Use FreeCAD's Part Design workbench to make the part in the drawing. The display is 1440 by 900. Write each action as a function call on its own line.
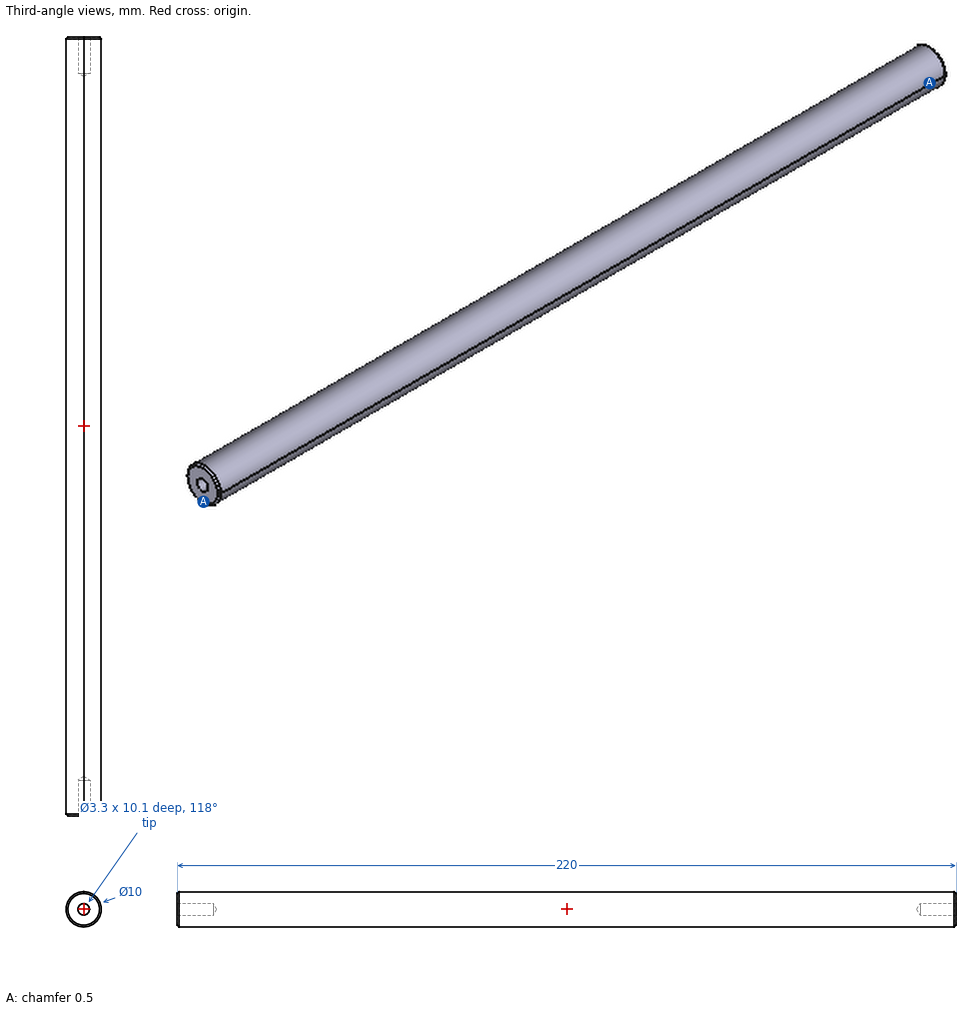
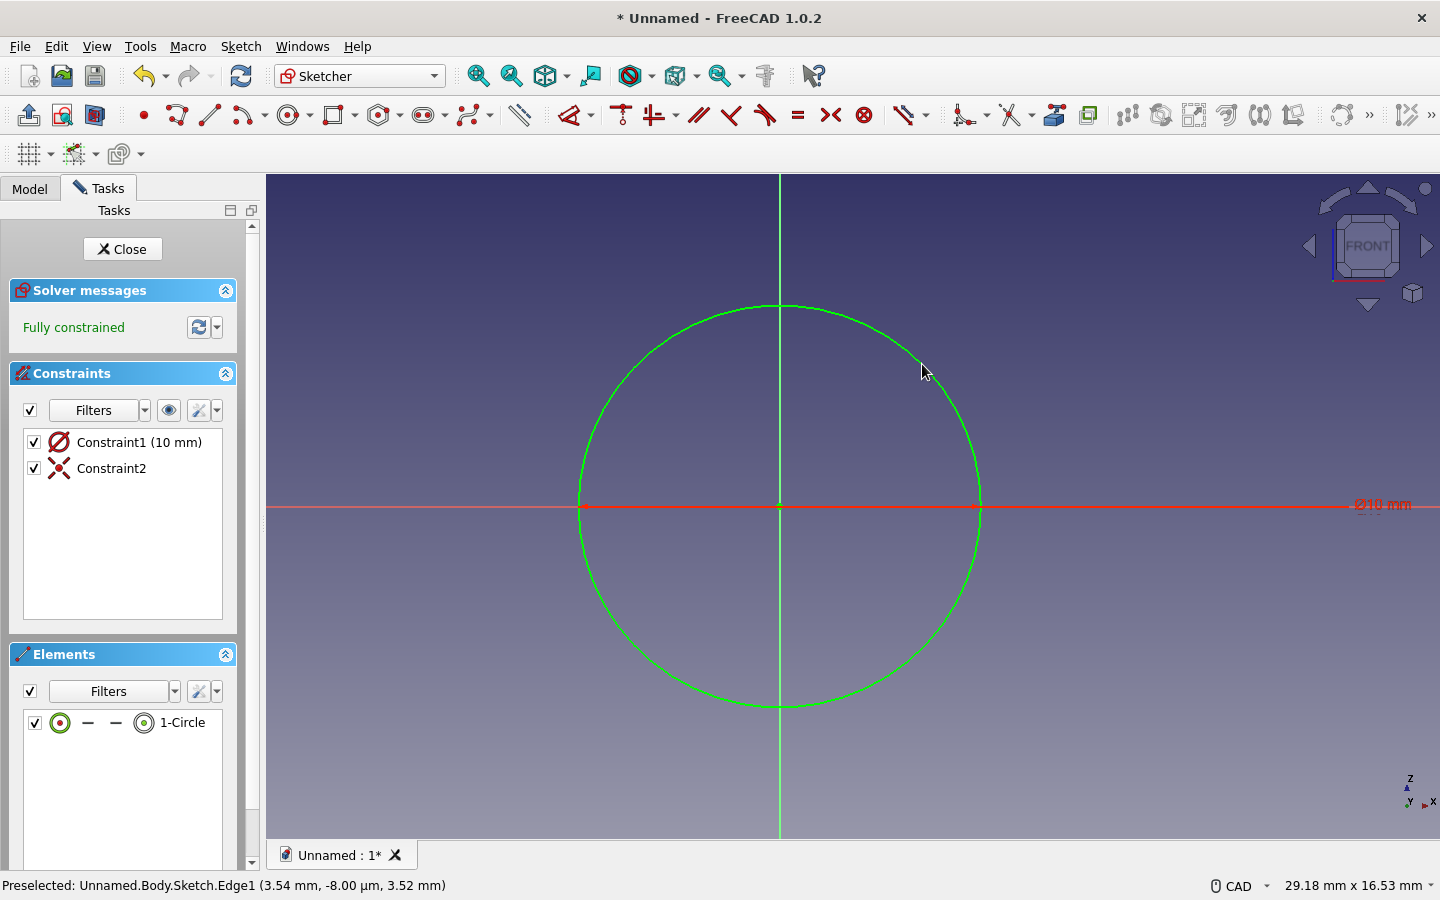
click(123, 249)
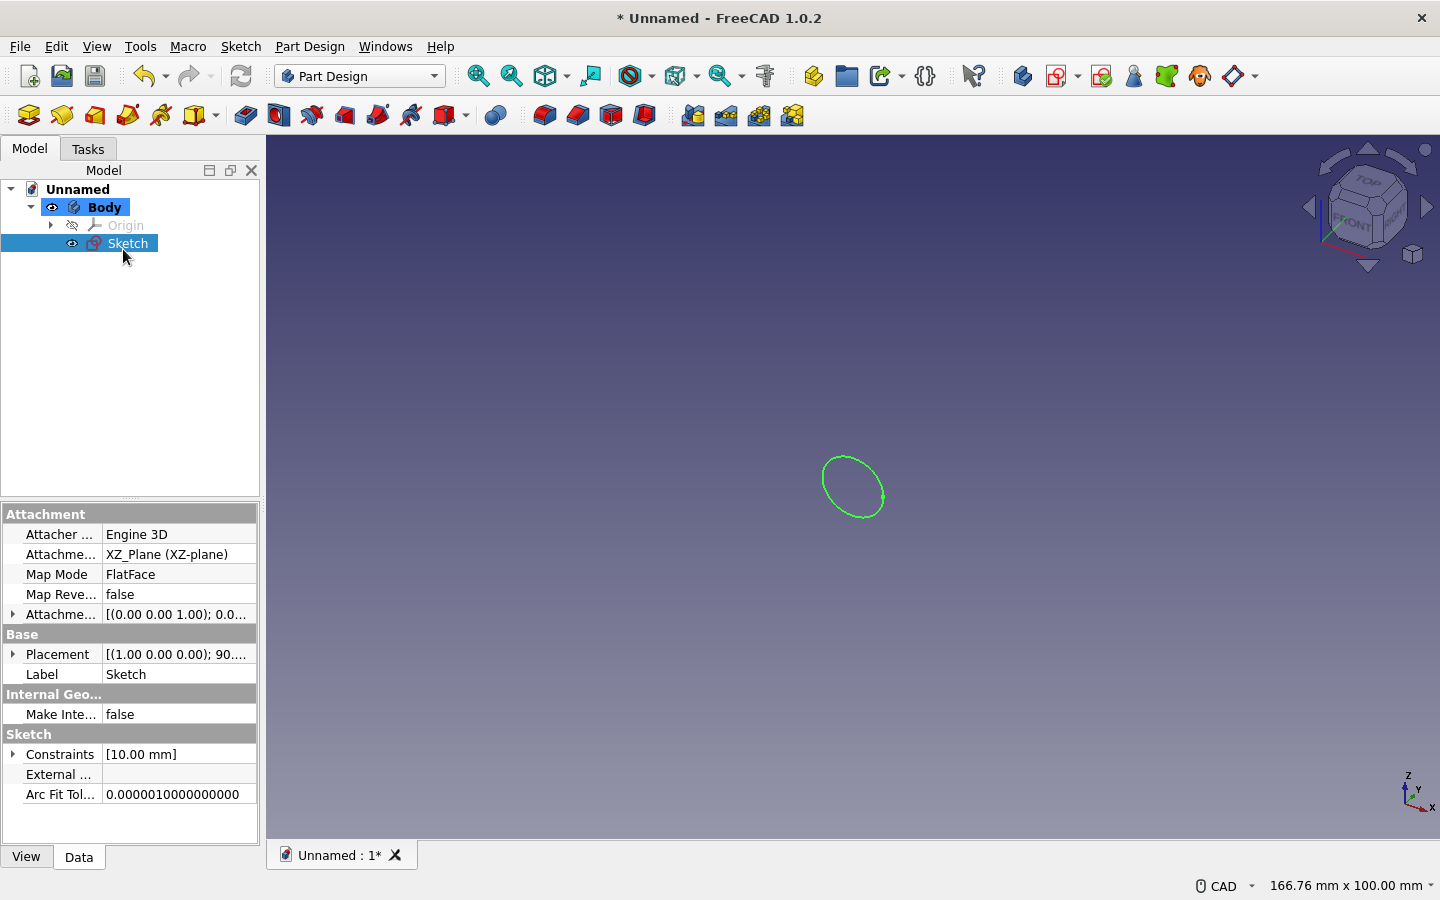
click(29, 116)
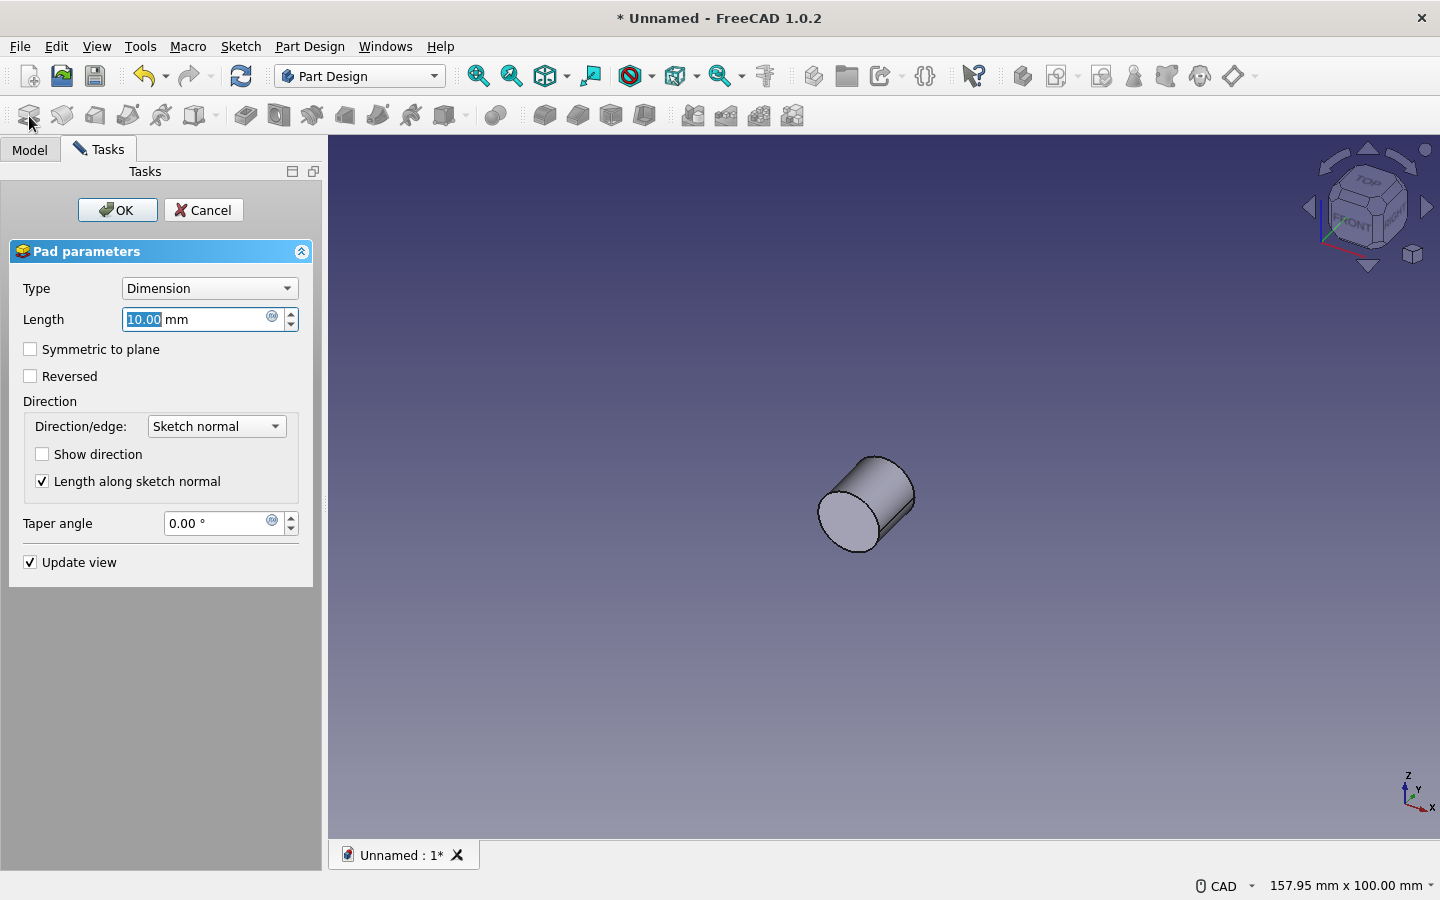
text(220)
key(Tab)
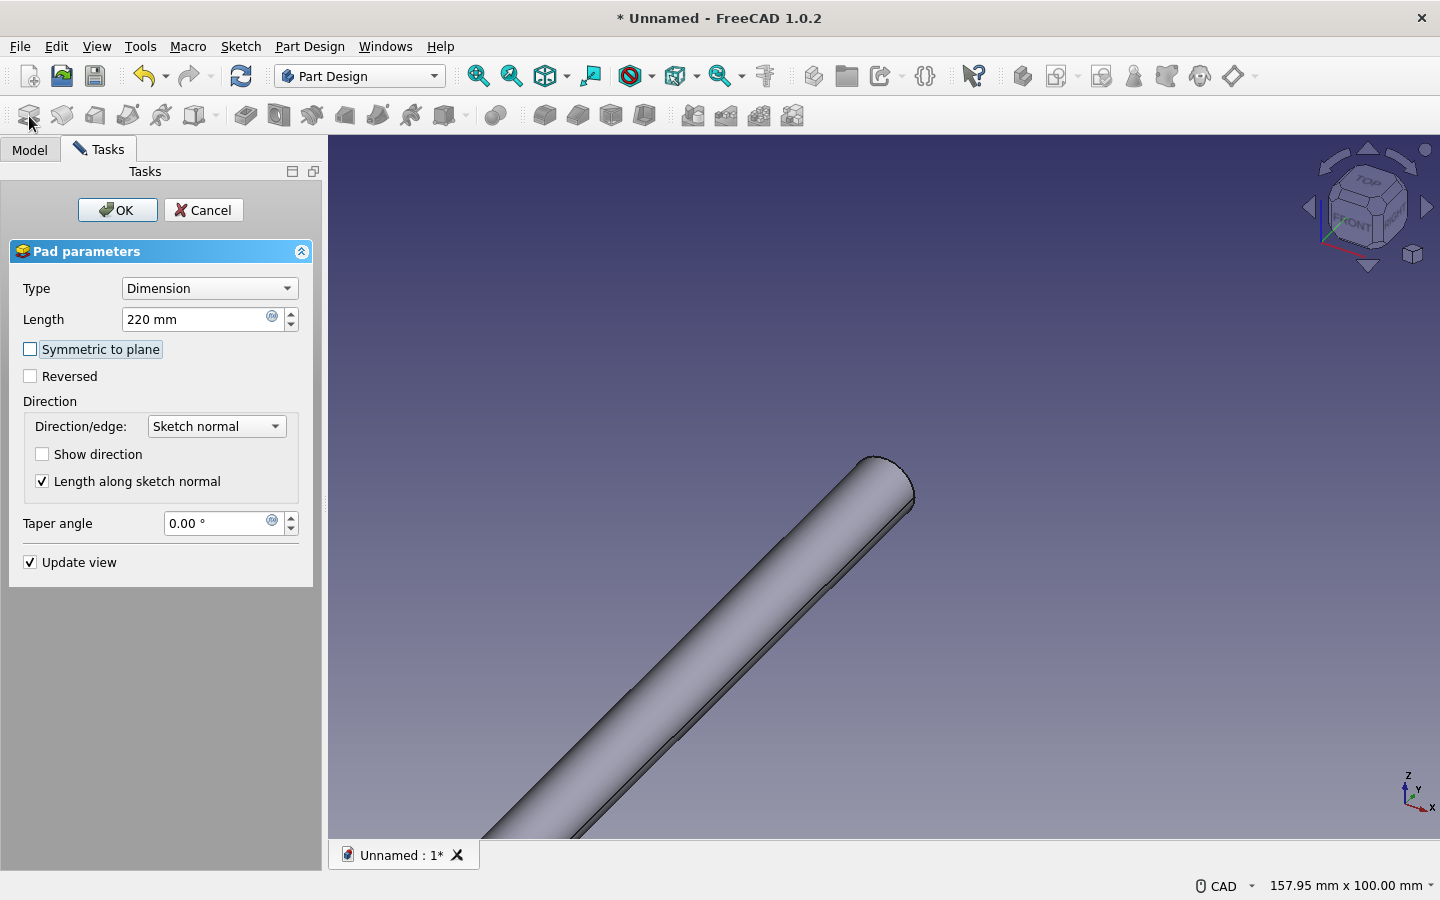
click(31, 349)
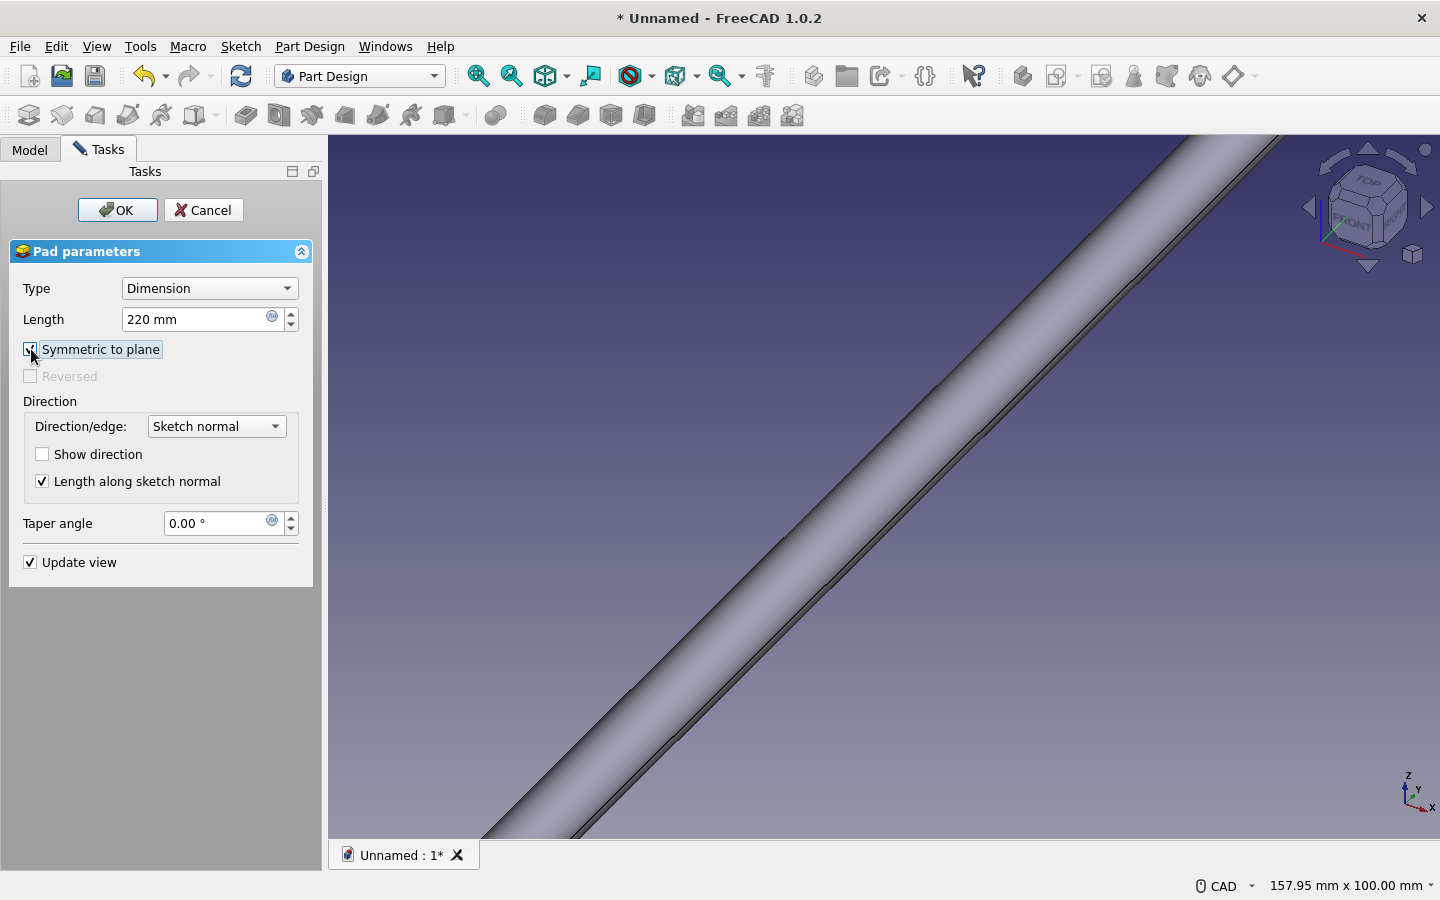
click(118, 210)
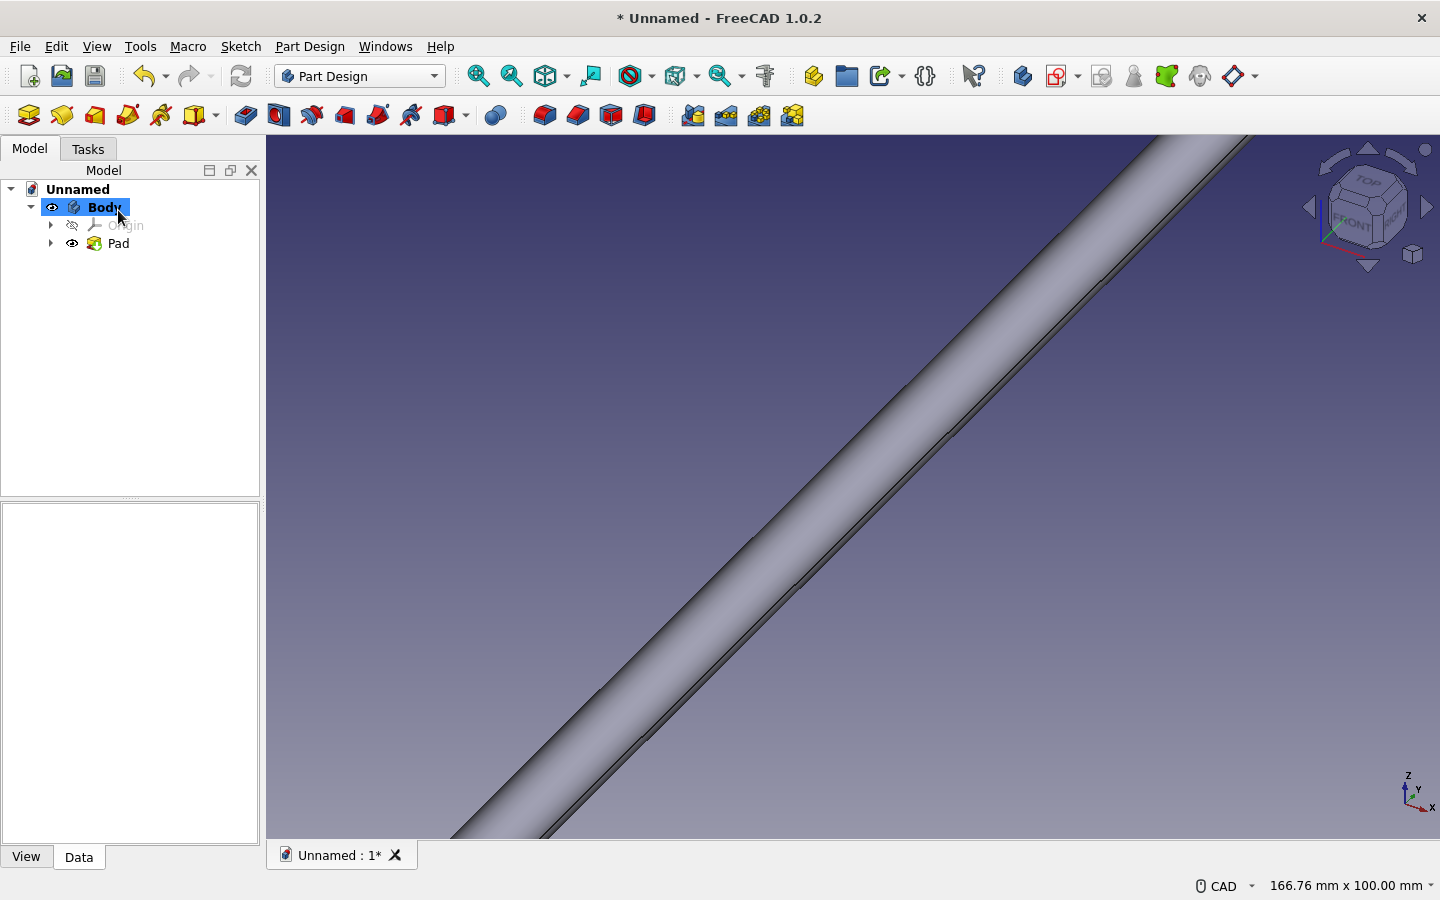
key(v)
key(f)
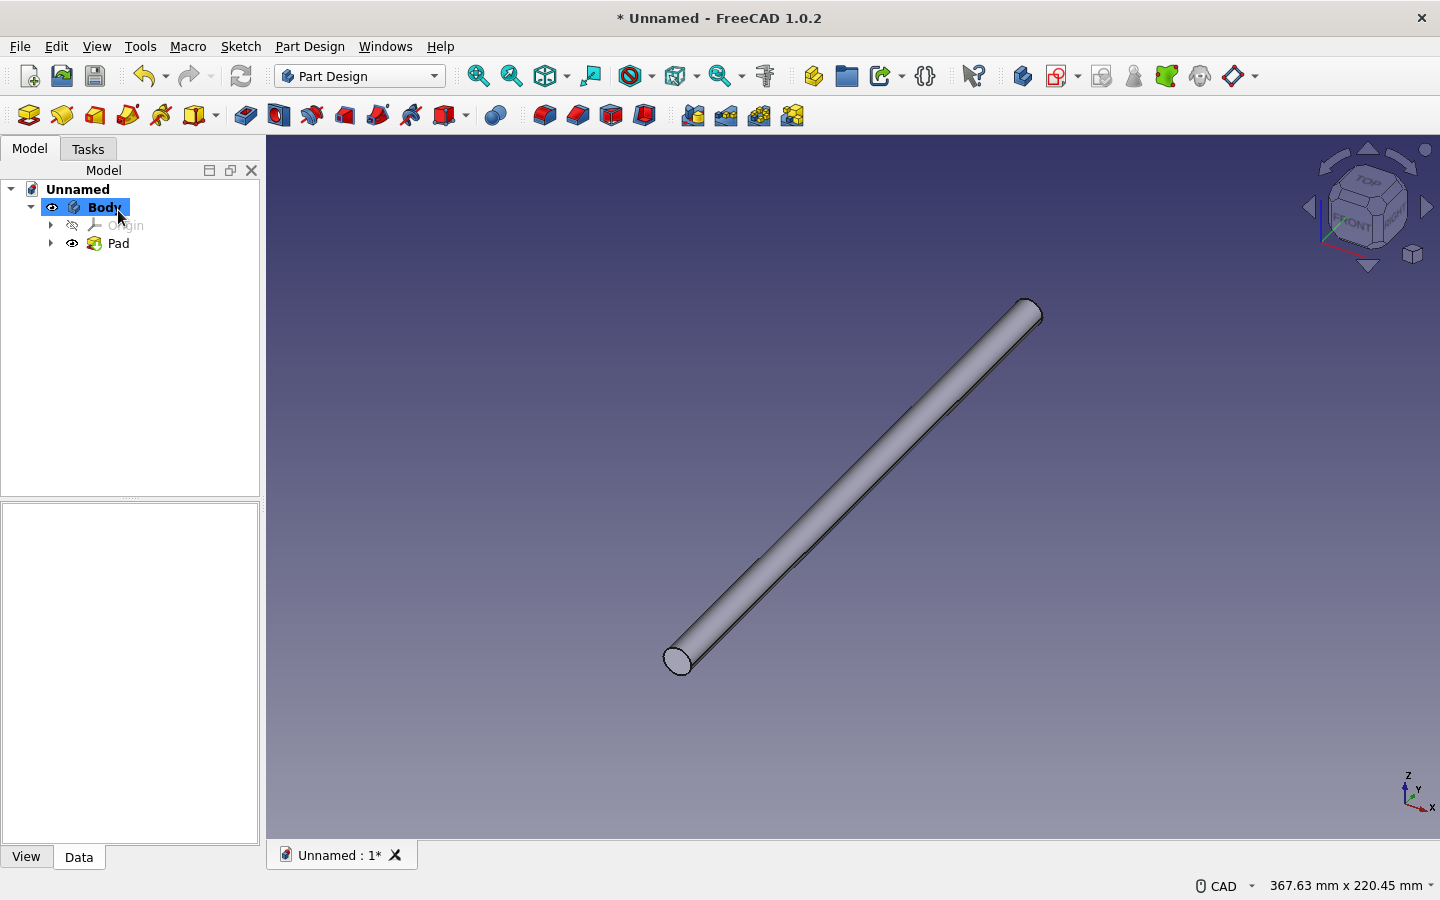
click(666, 649)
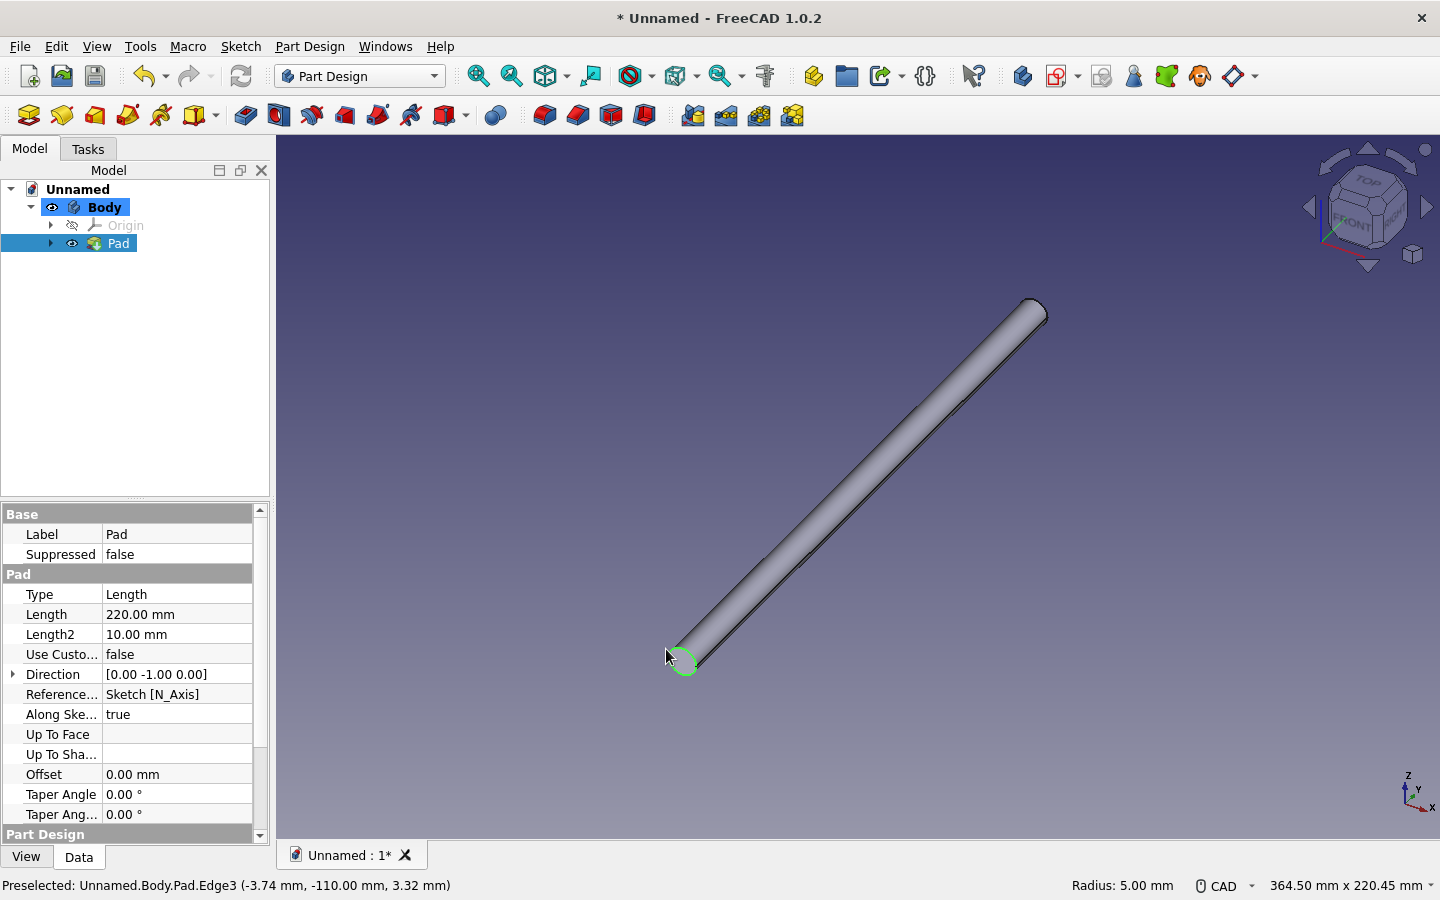
key(0)